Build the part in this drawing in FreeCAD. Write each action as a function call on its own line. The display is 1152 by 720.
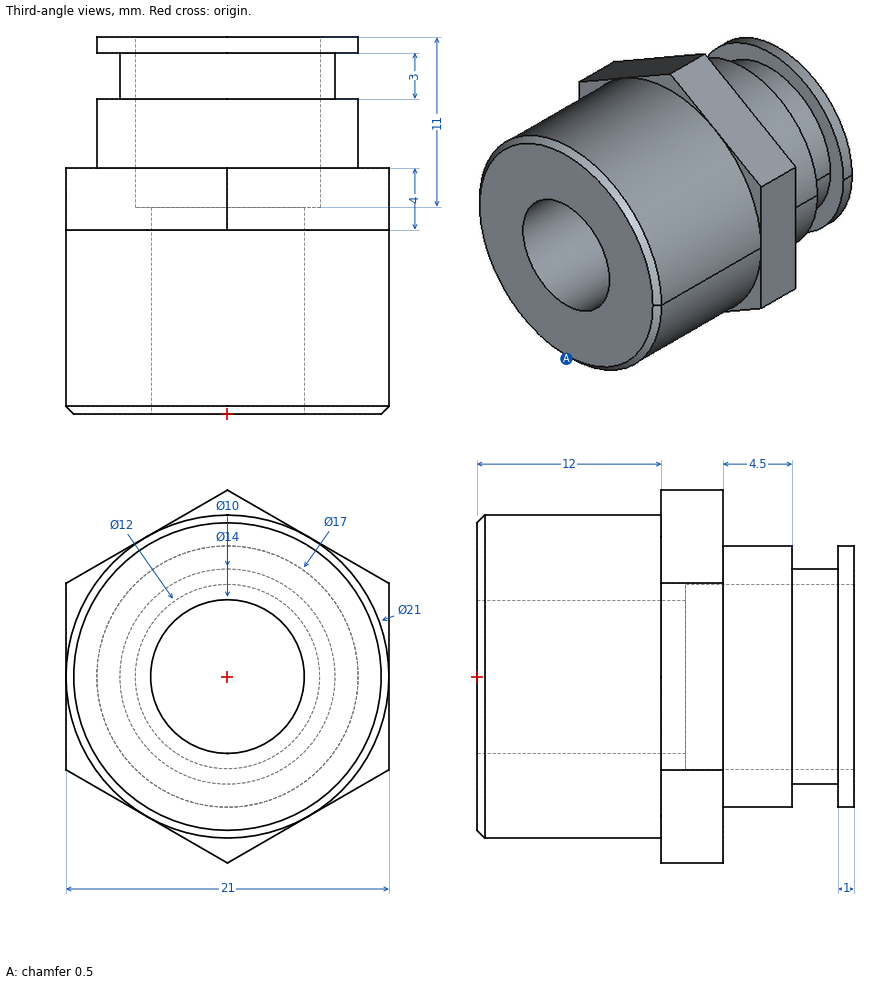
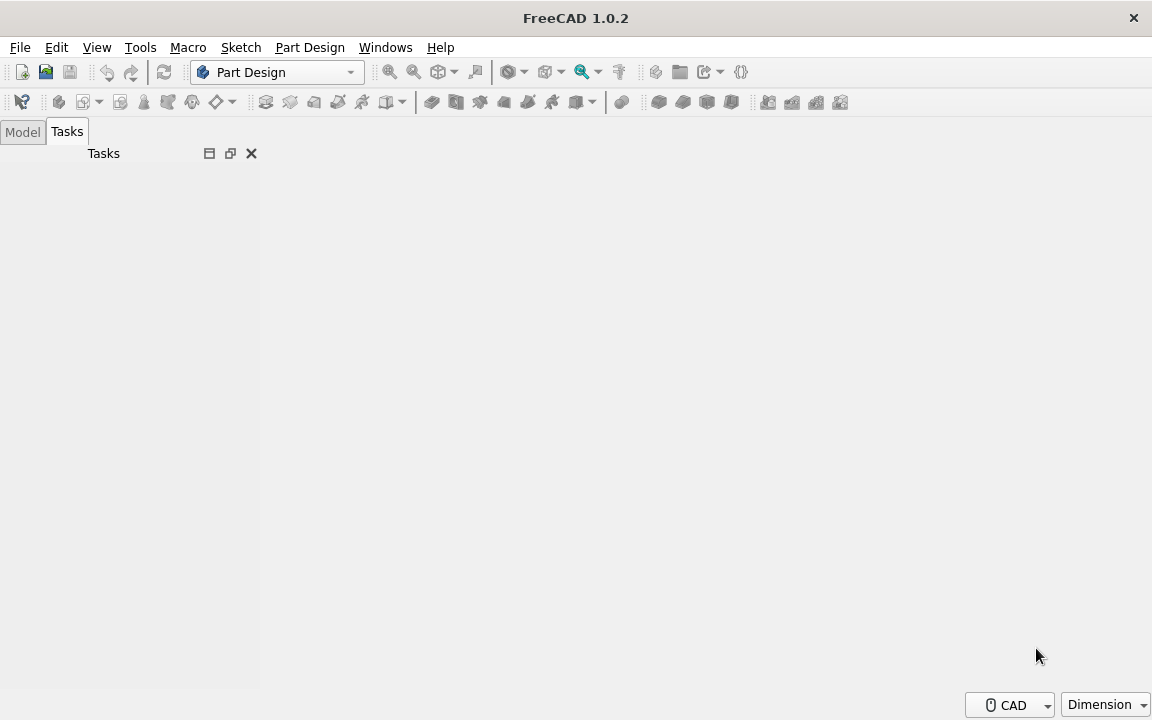
click(22, 72)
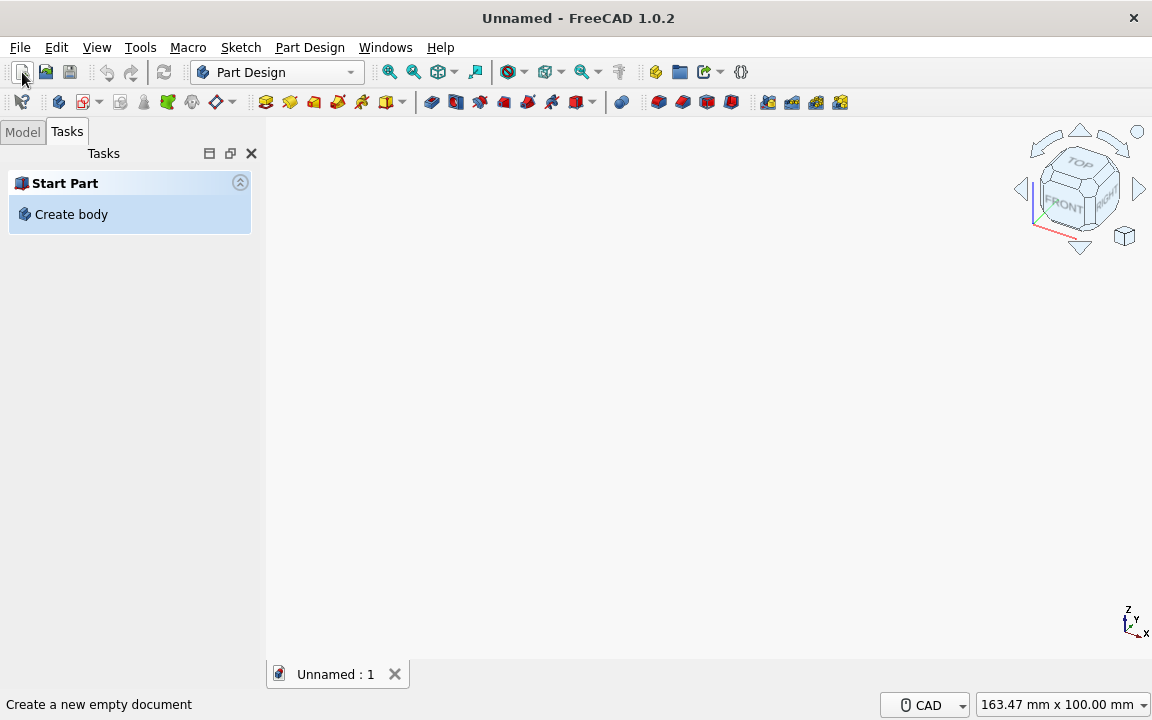
click(84, 102)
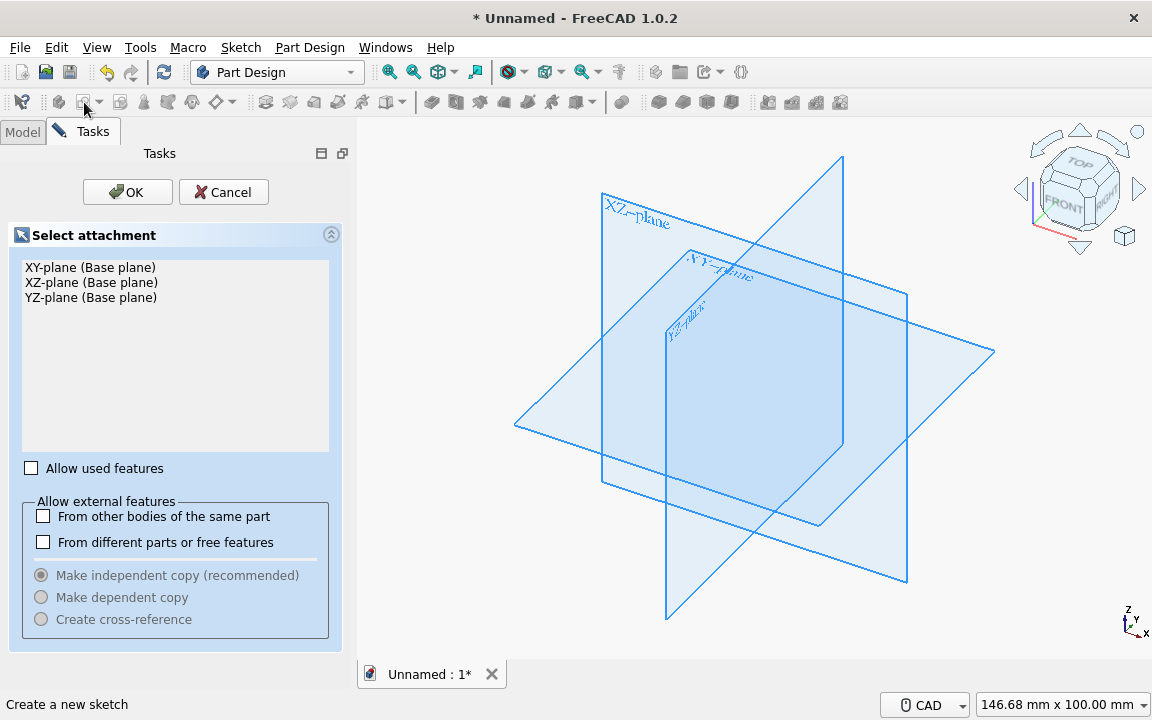
click(82, 282)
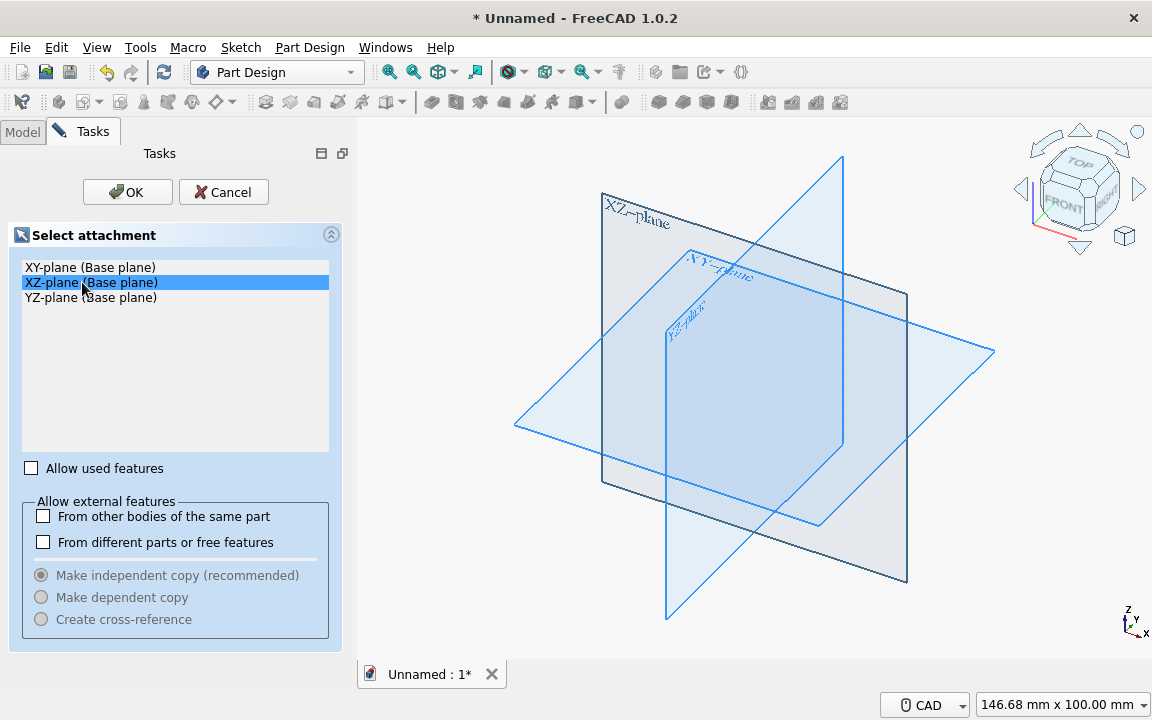
click(128, 192)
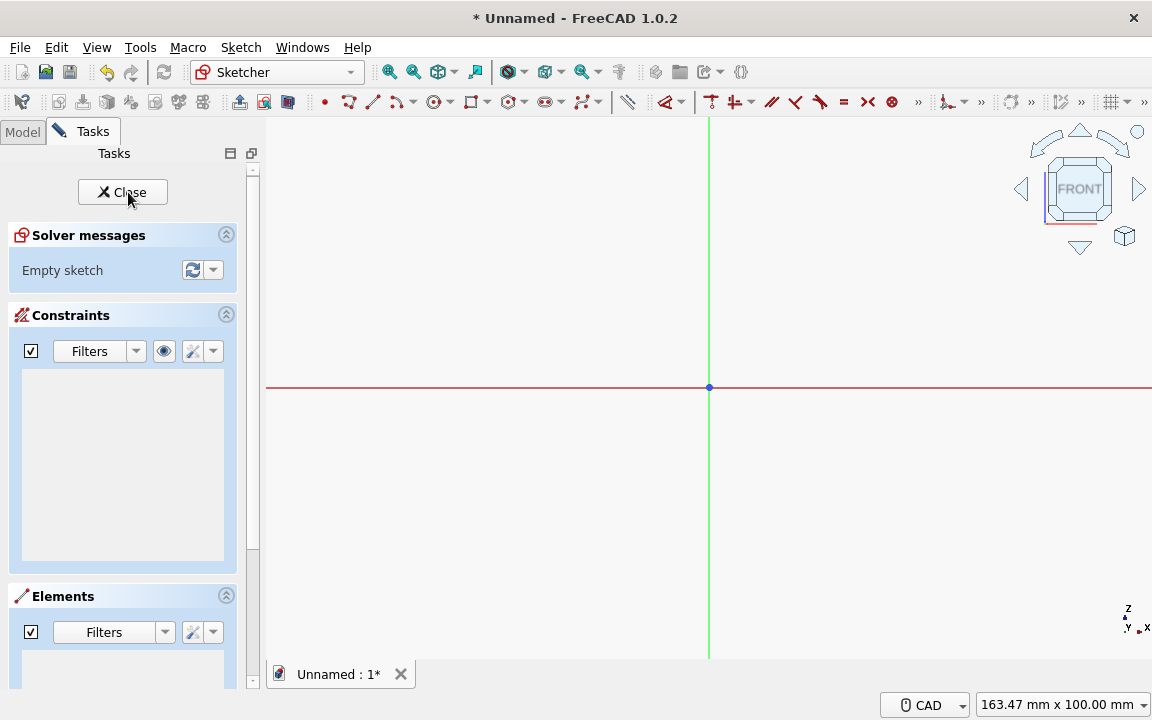
scroll(739, 388, up, 6)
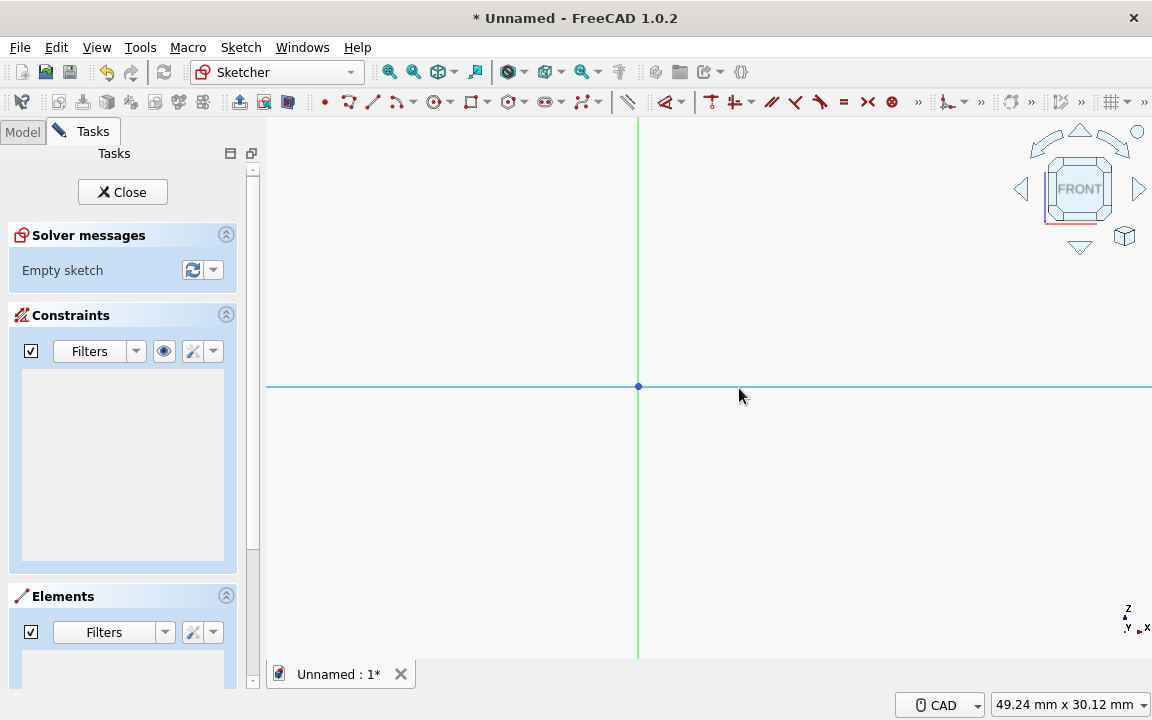
key(g)
key(c)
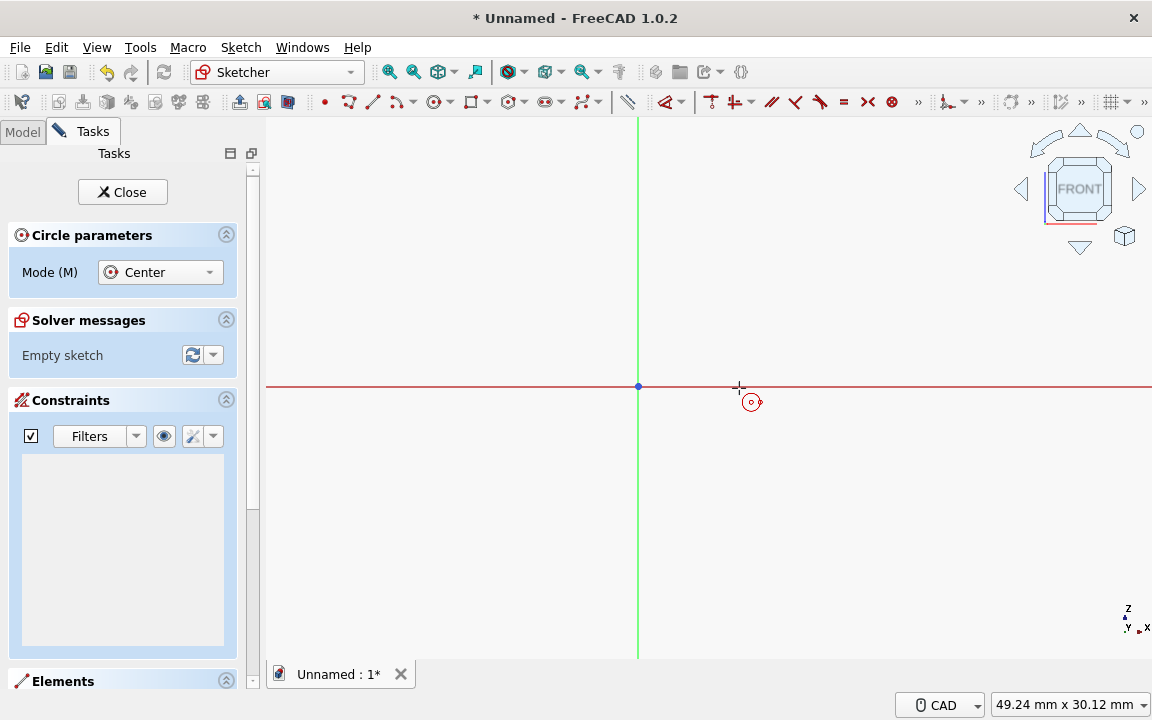
click(638, 387)
move(772, 253)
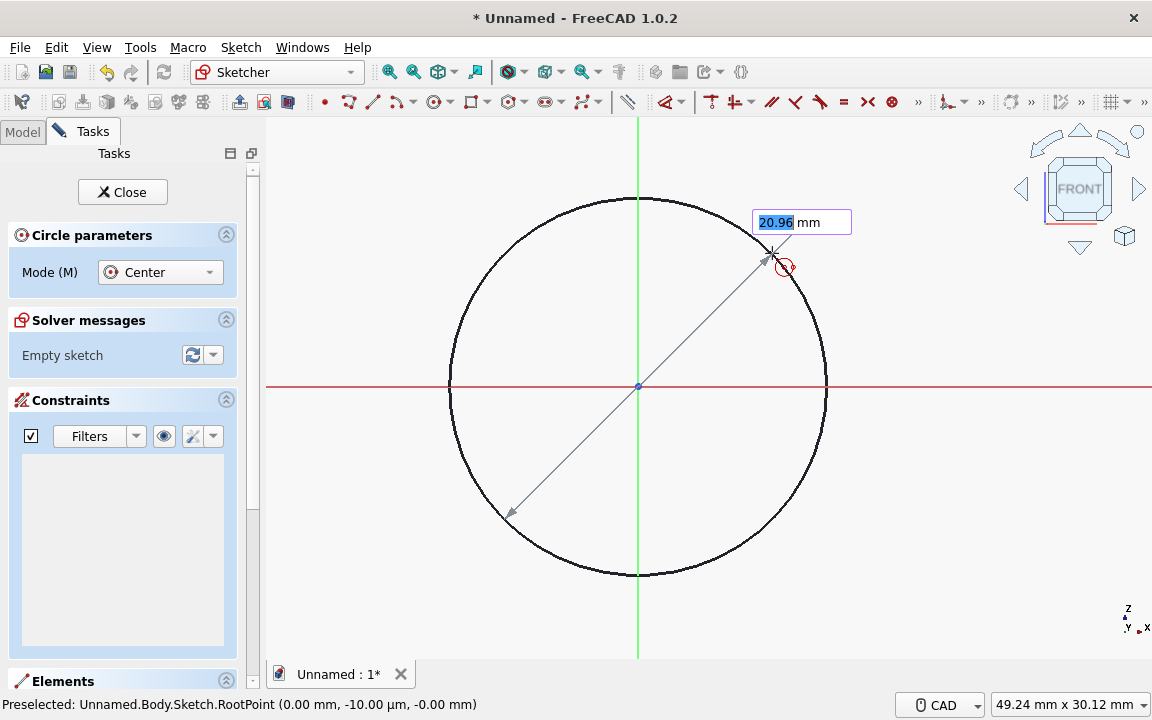
text(21)
key(Return)
key(Escape)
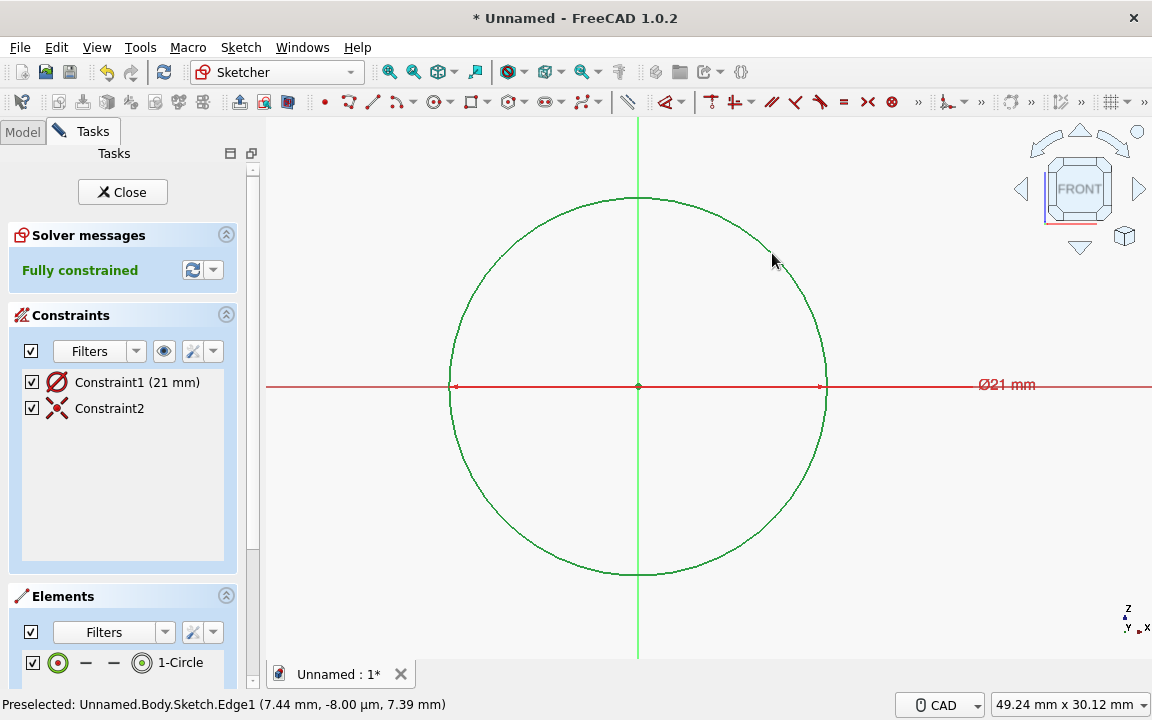
click(123, 192)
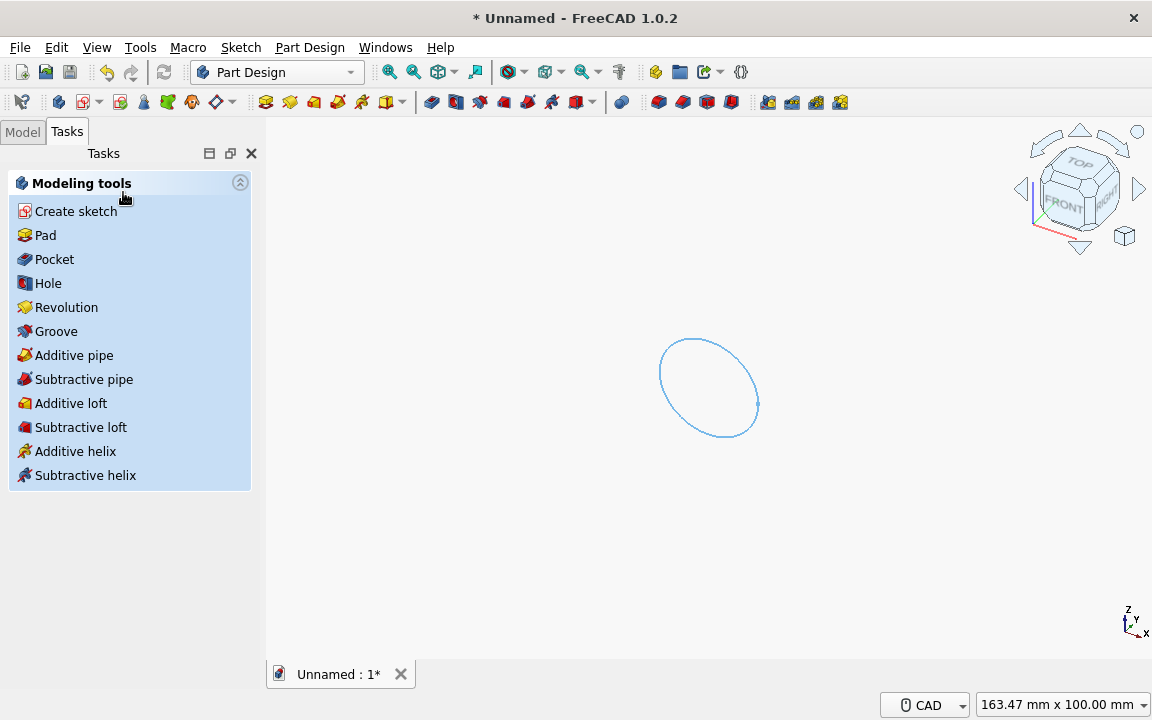
click(266, 102)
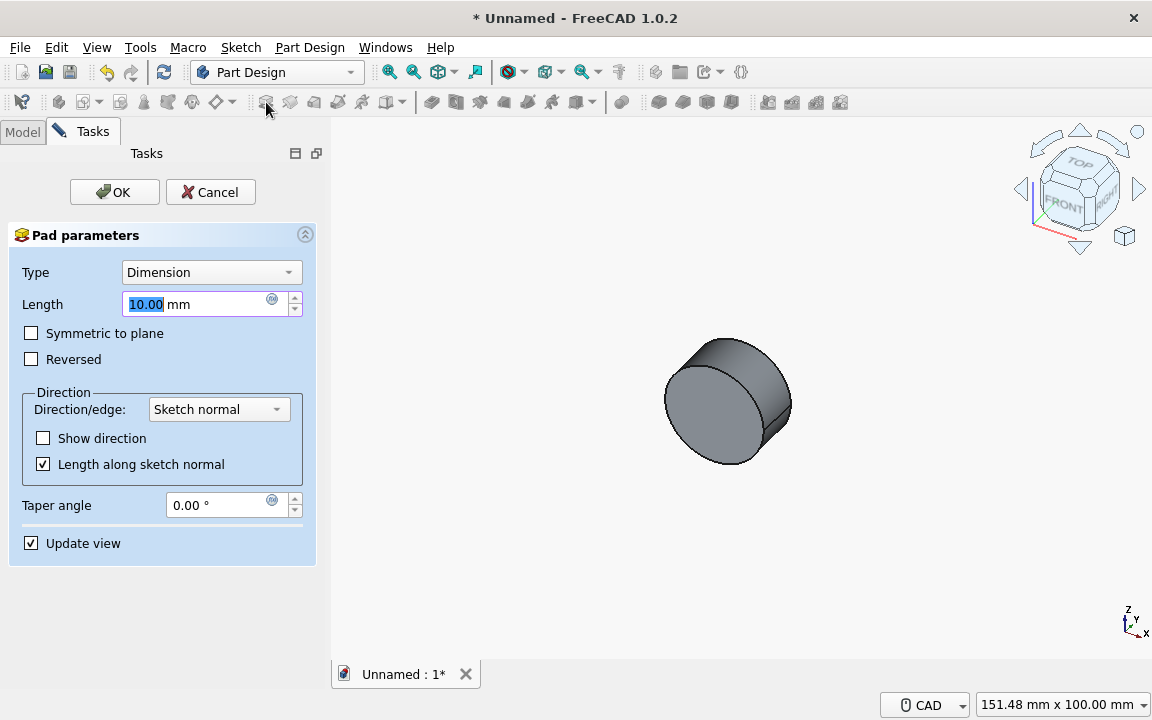
text(12)
key(Tab)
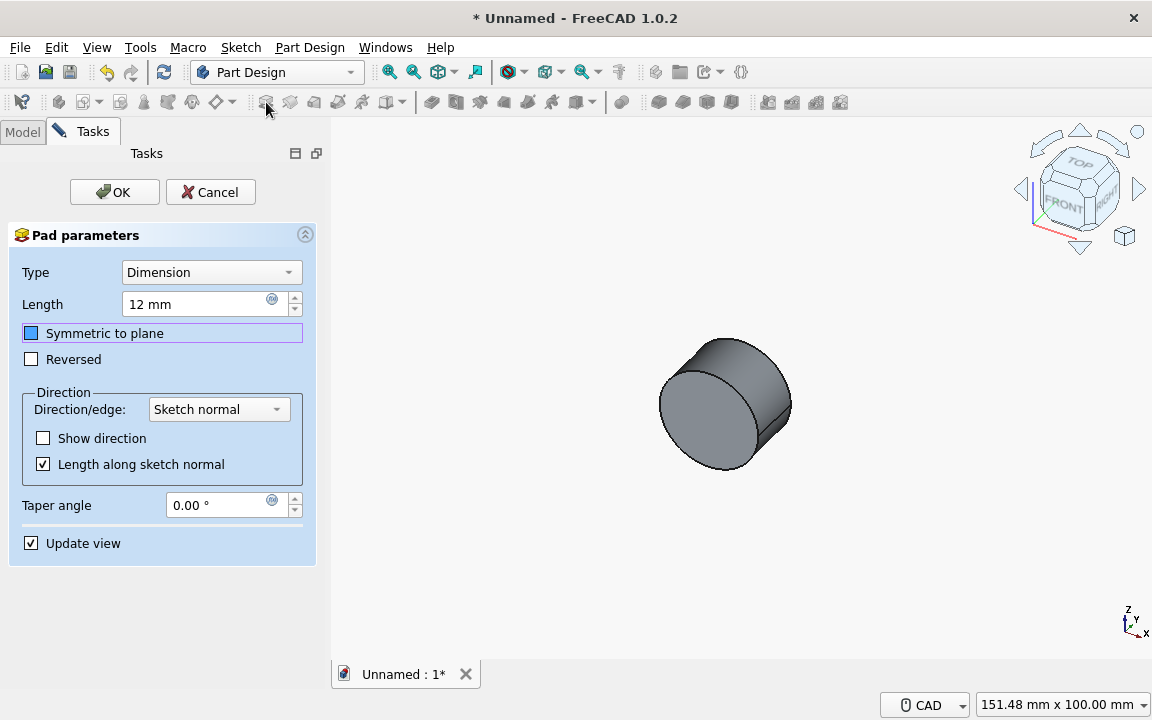
click(30, 359)